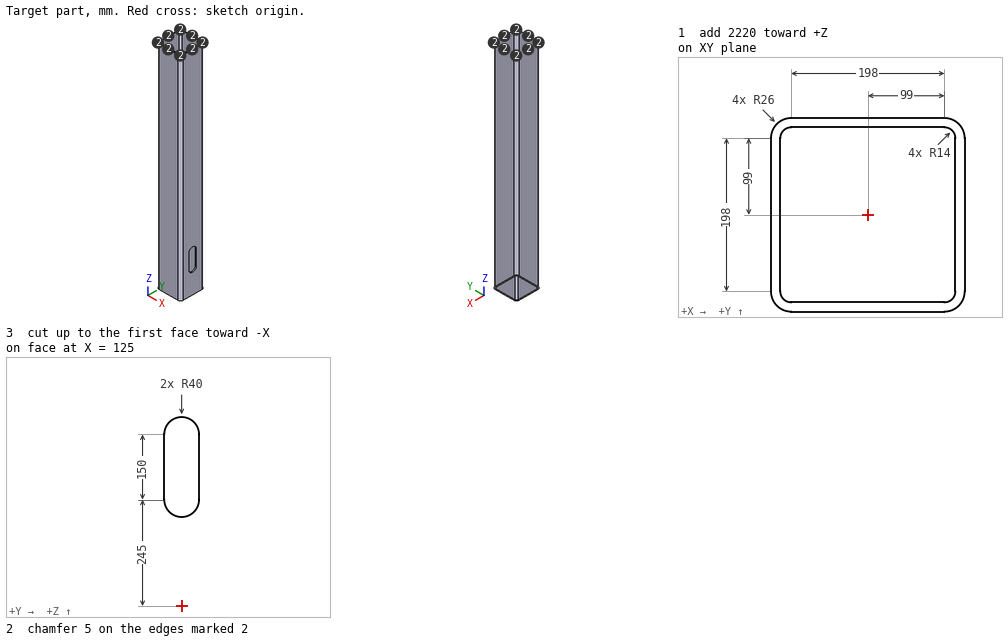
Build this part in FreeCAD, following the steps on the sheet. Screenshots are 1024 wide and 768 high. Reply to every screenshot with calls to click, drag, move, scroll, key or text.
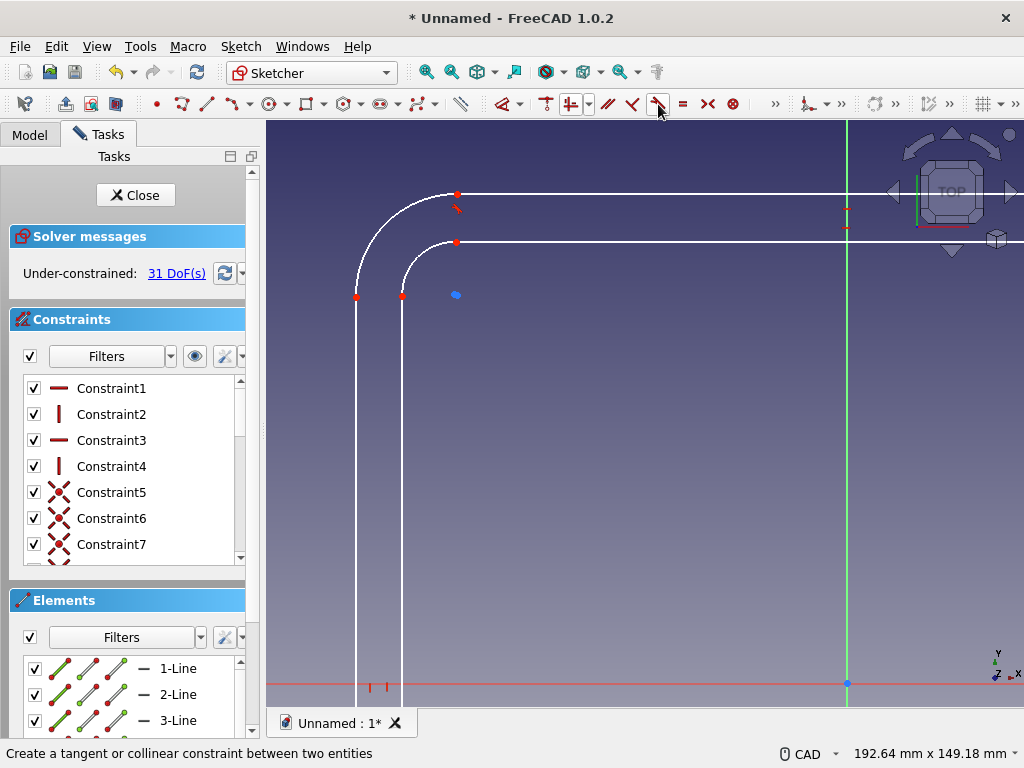
click(691, 194)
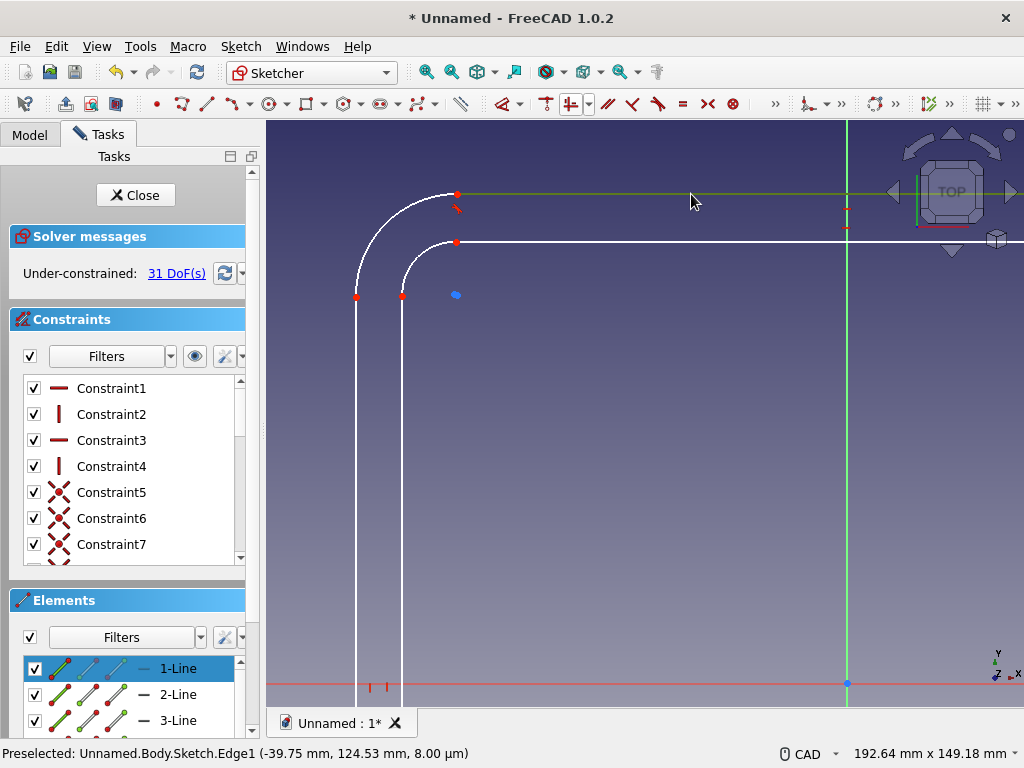
scroll(419, 256, down, 5)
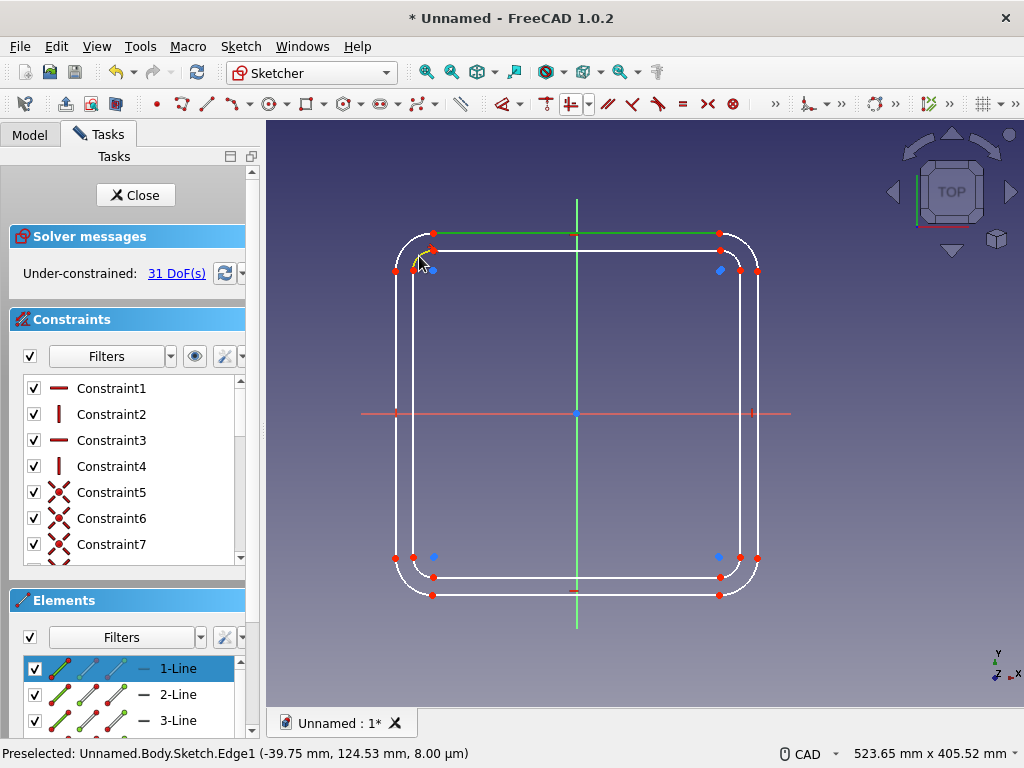
click(754, 254)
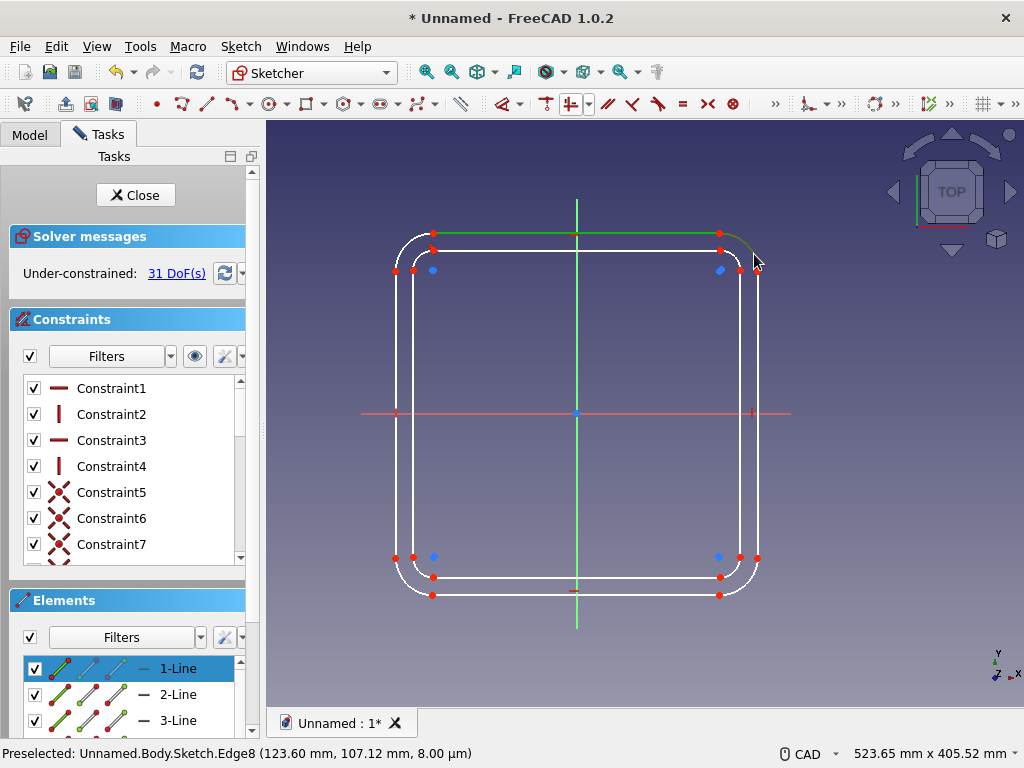
click(658, 104)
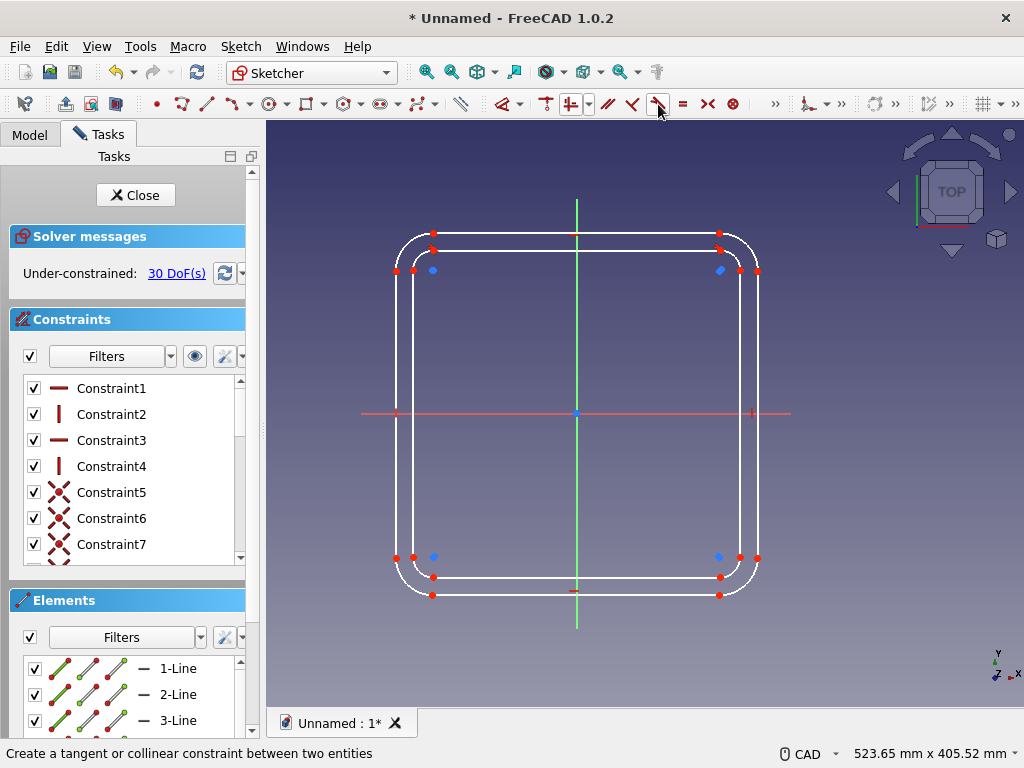
click(396, 357)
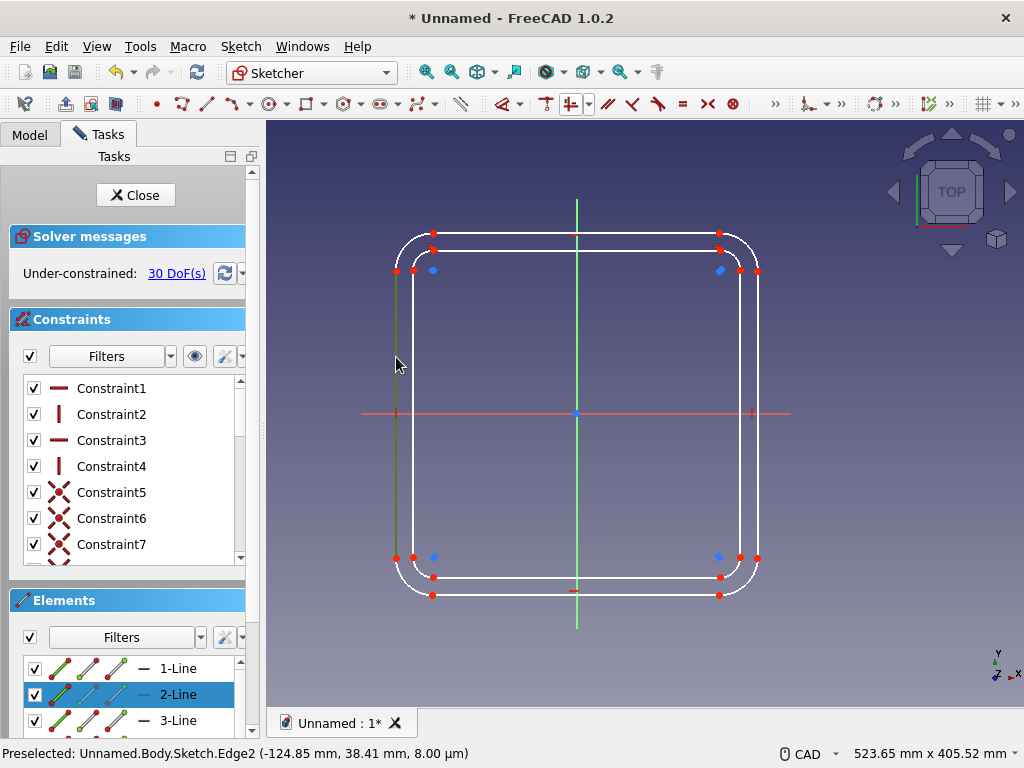
click(416, 238)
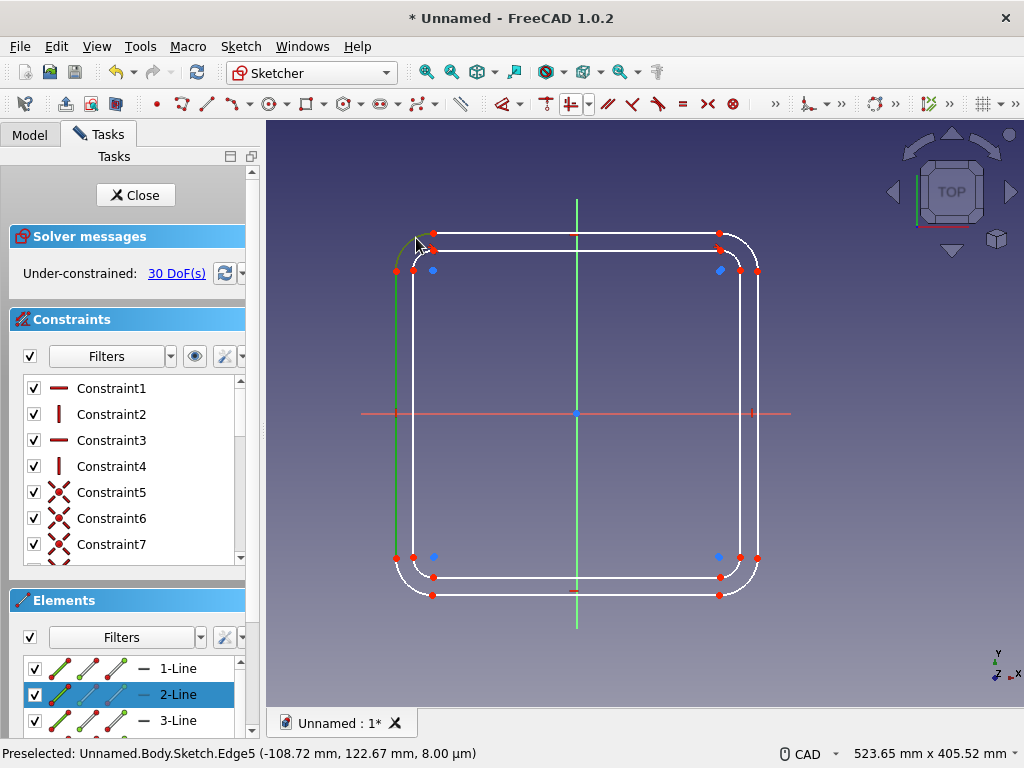
click(658, 104)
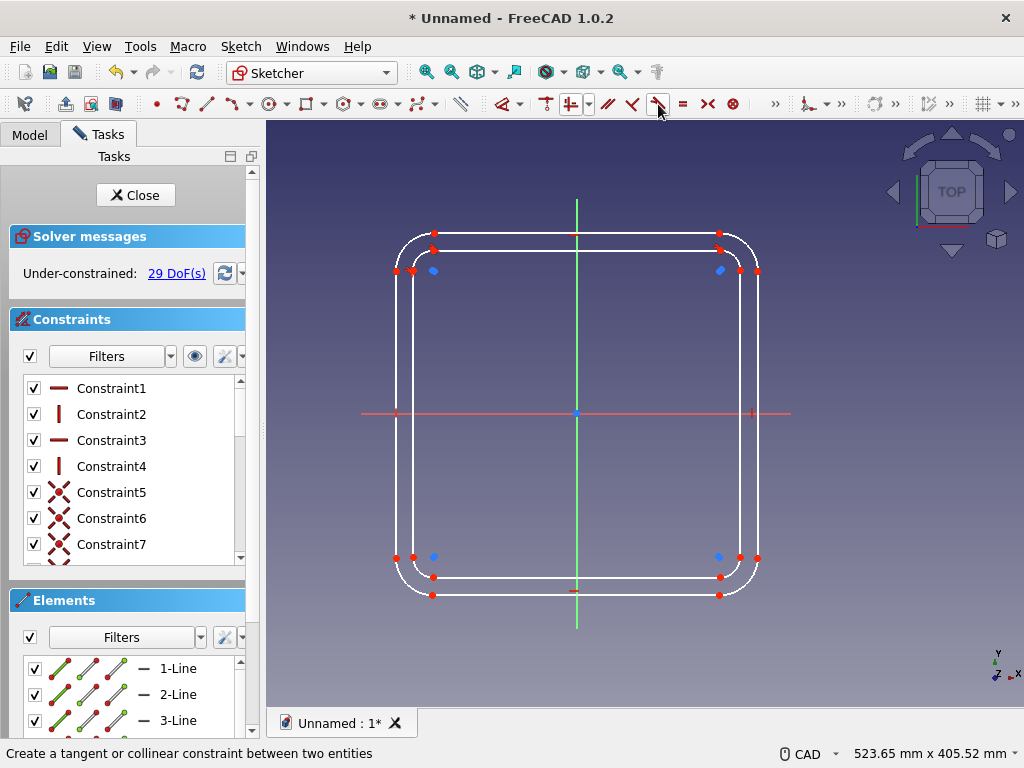
click(396, 357)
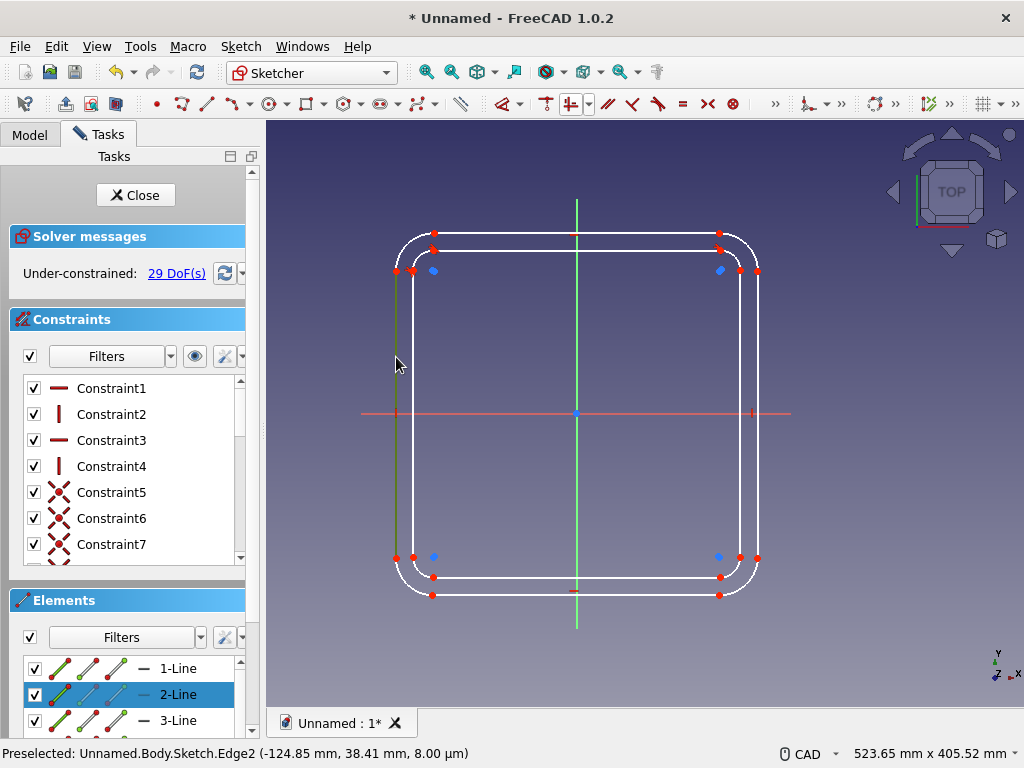
click(400, 575)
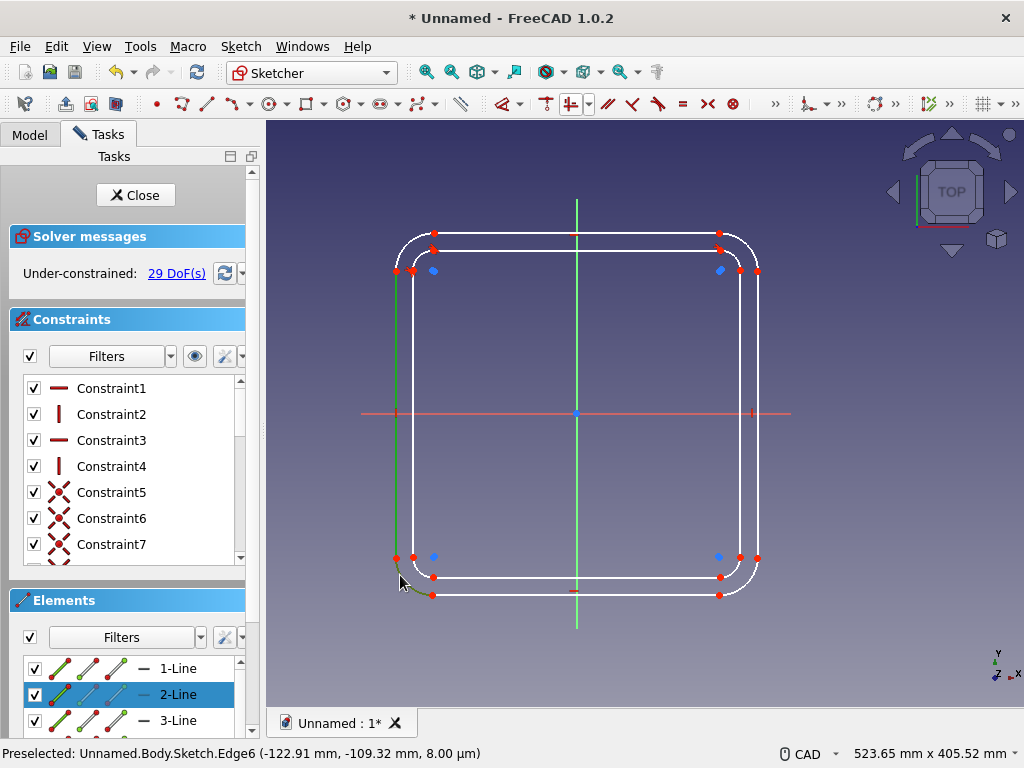
click(658, 104)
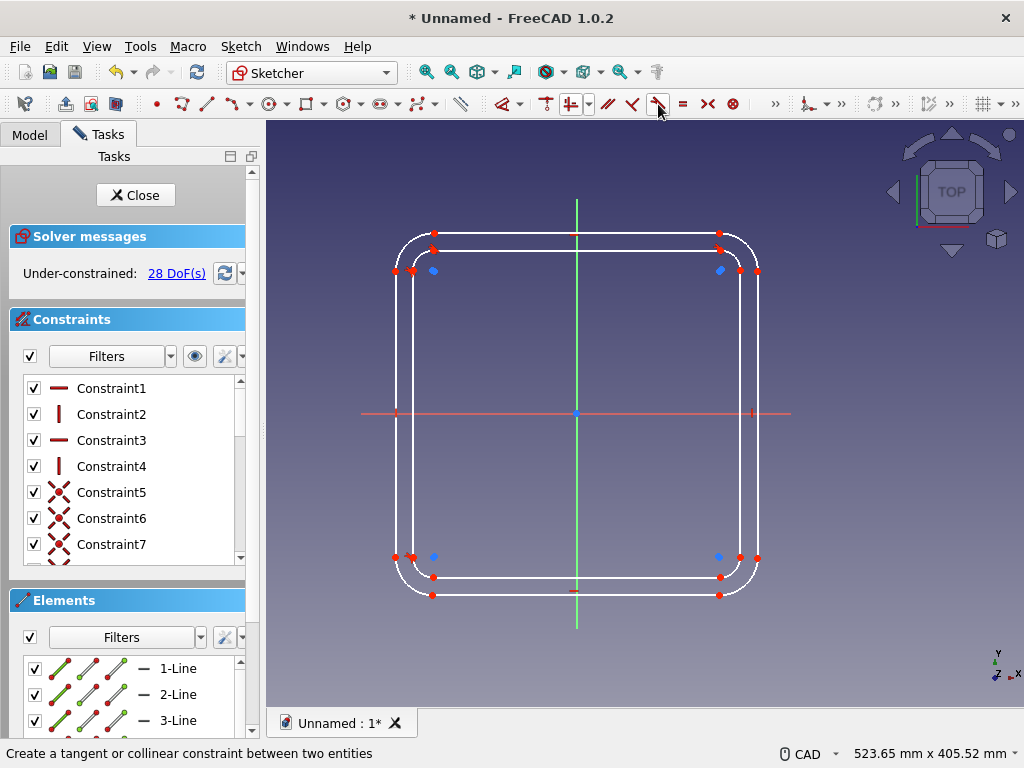
click(519, 595)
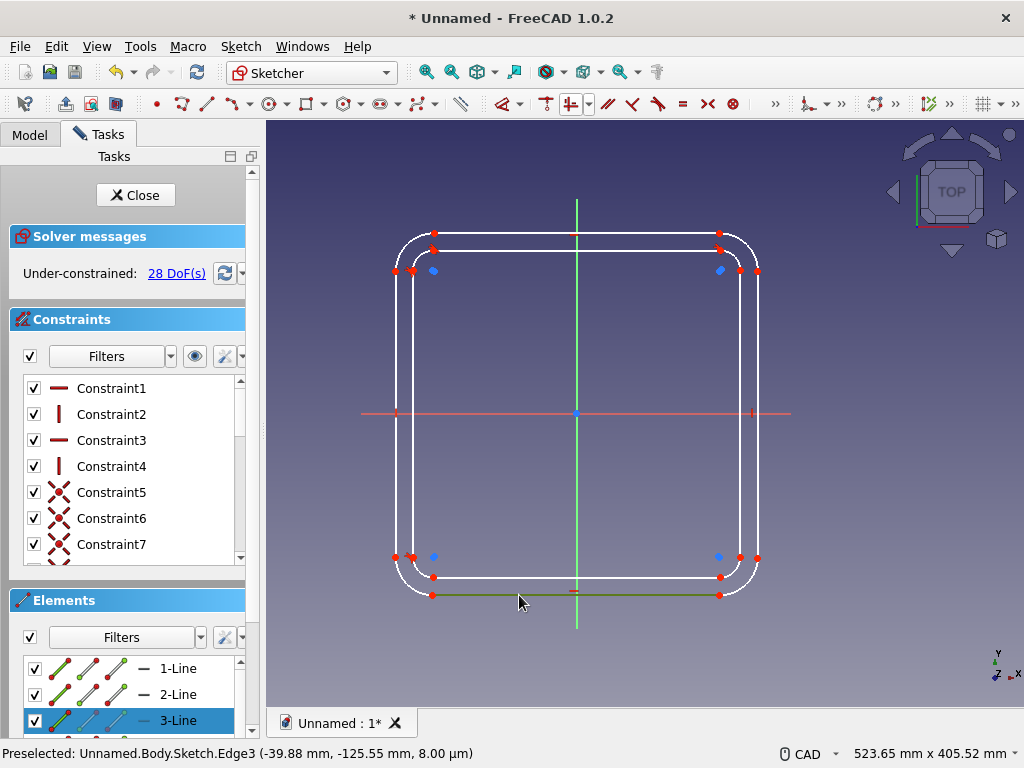
click(400, 574)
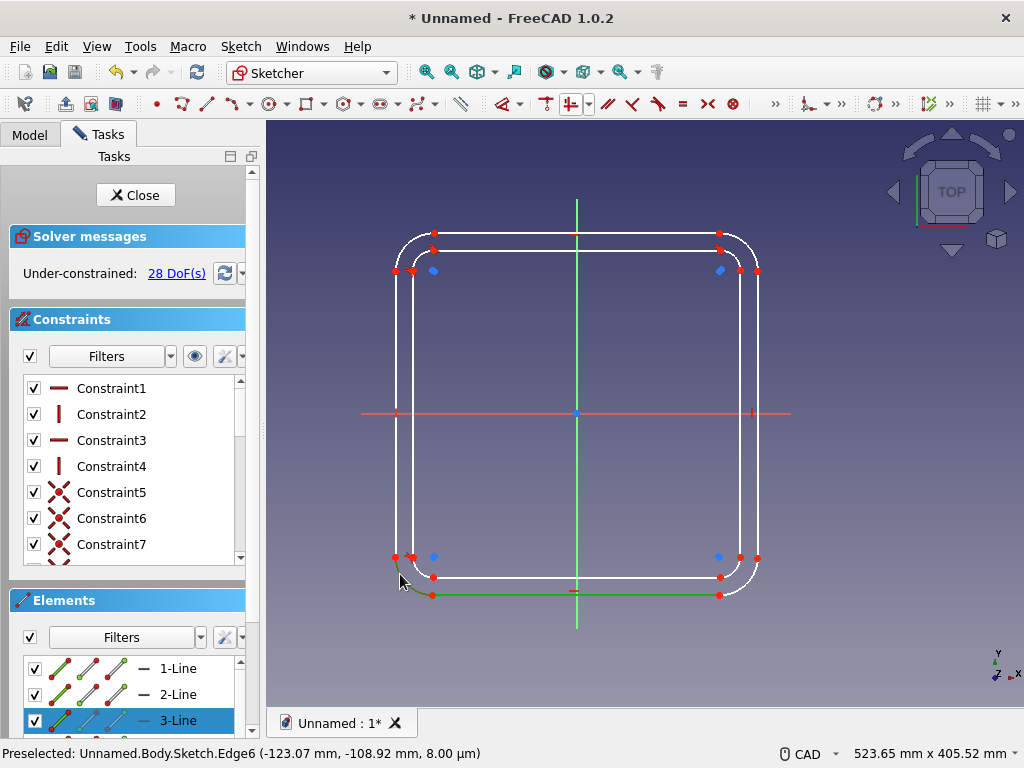
click(658, 104)